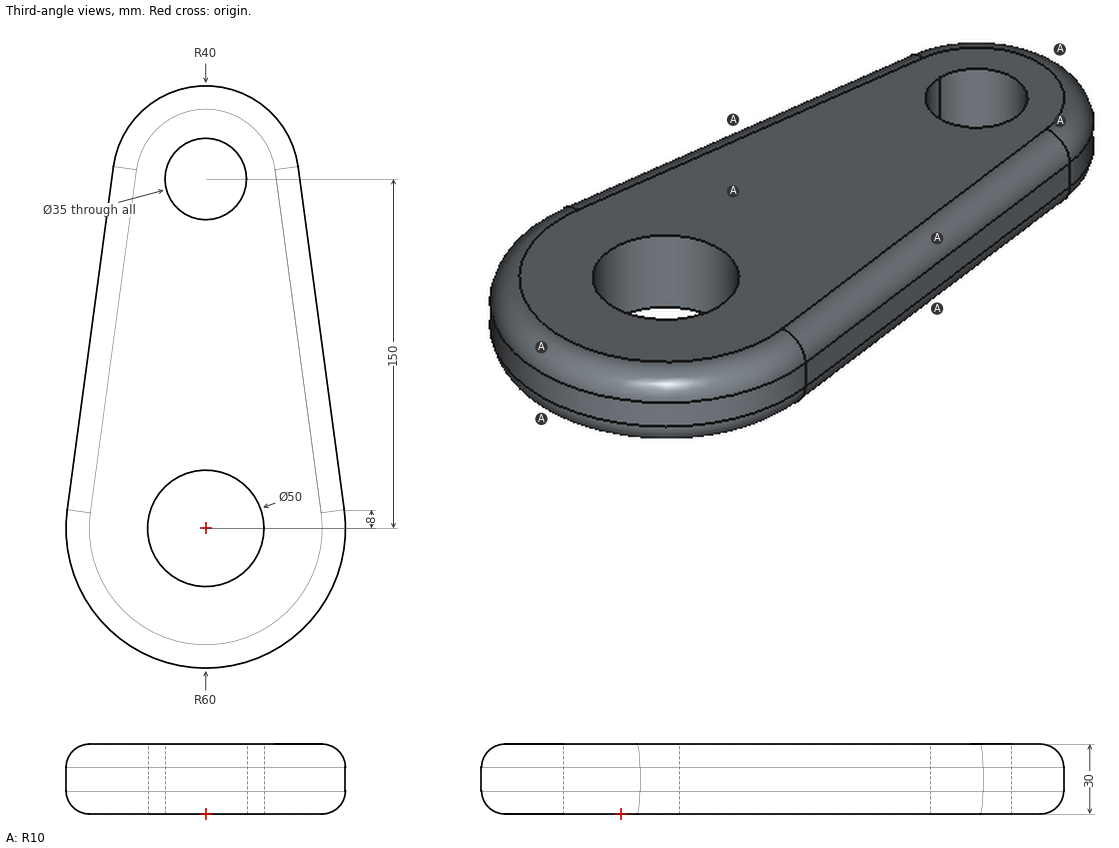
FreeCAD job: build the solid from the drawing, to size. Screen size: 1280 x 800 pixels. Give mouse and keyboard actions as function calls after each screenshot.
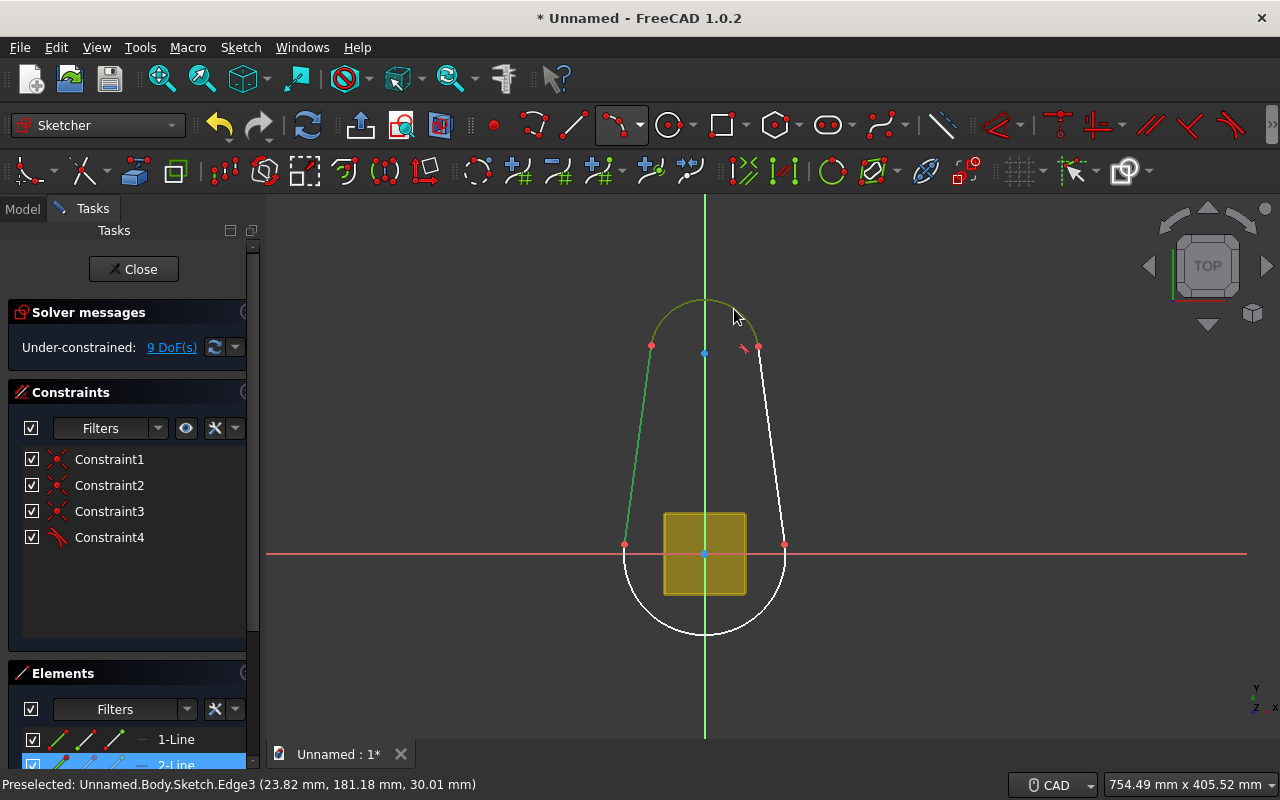
click(1232, 126)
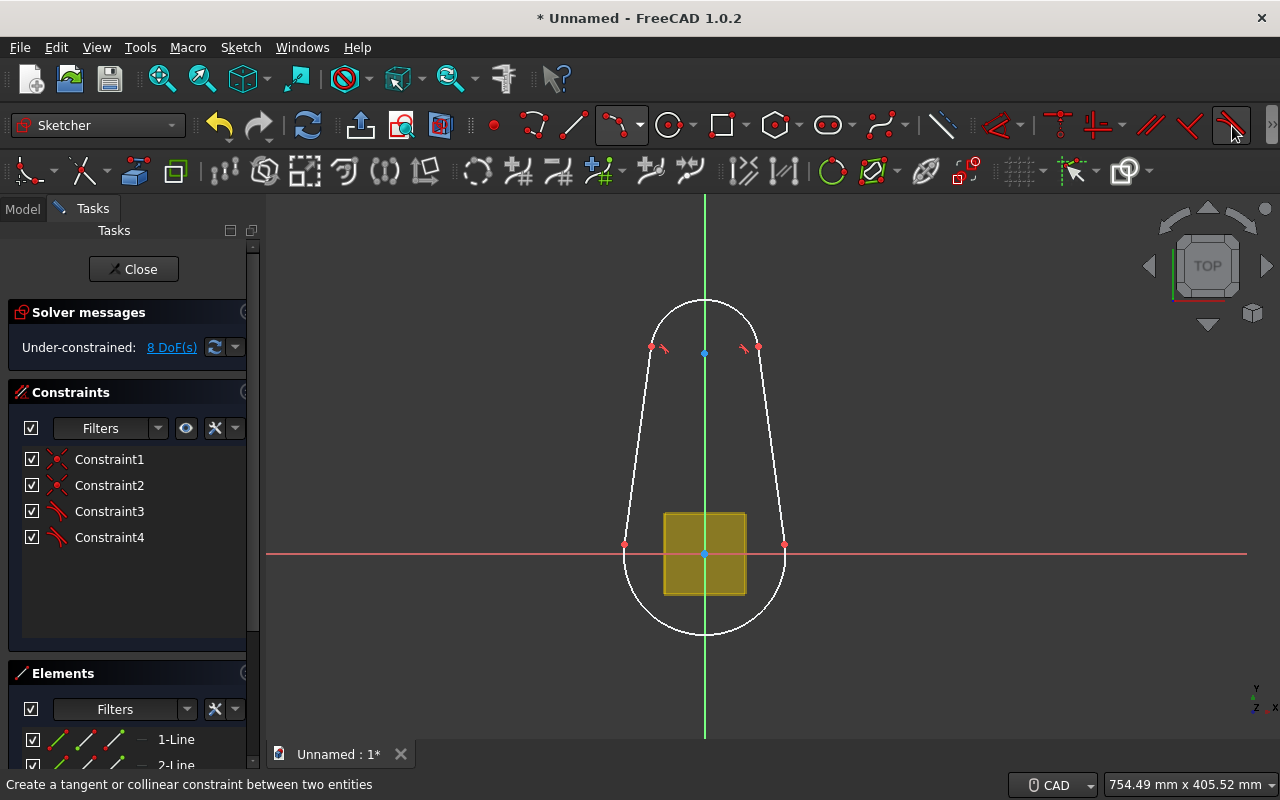
drag(695, 544, 715, 564)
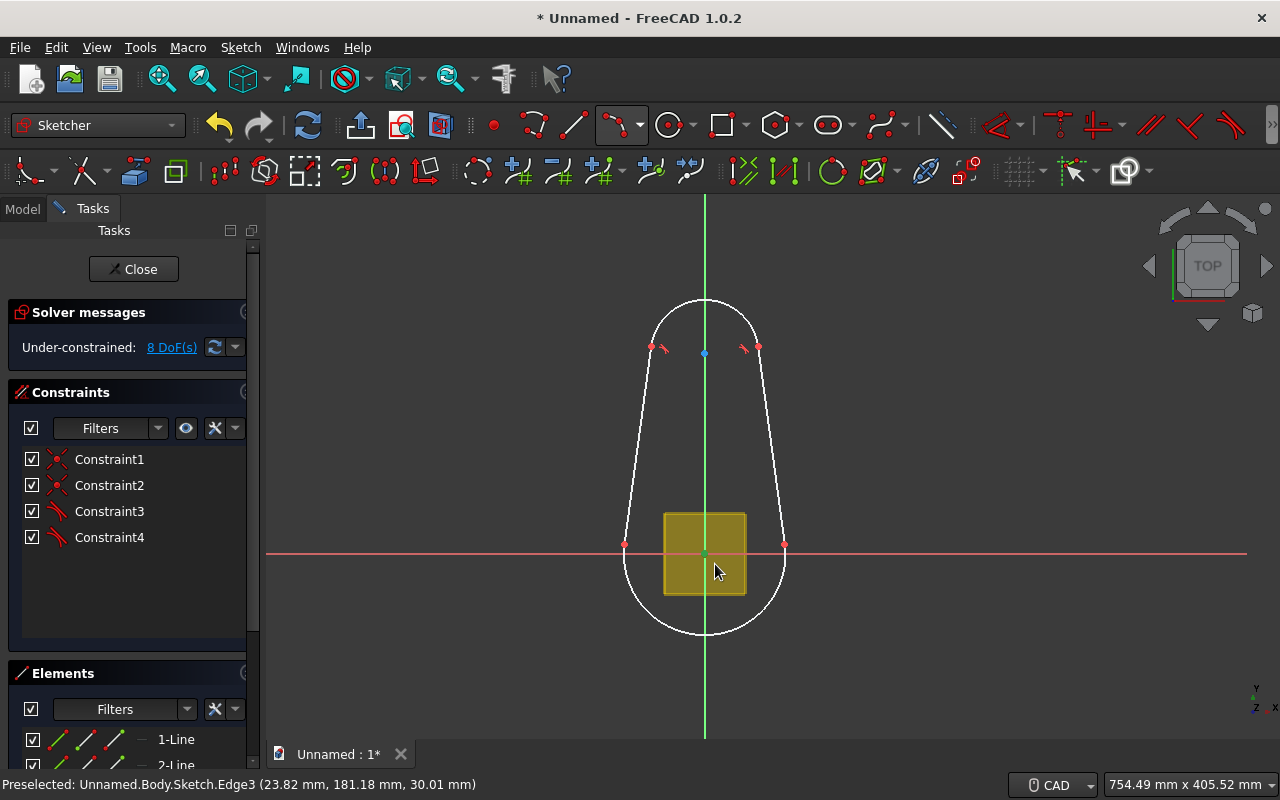
click(1058, 126)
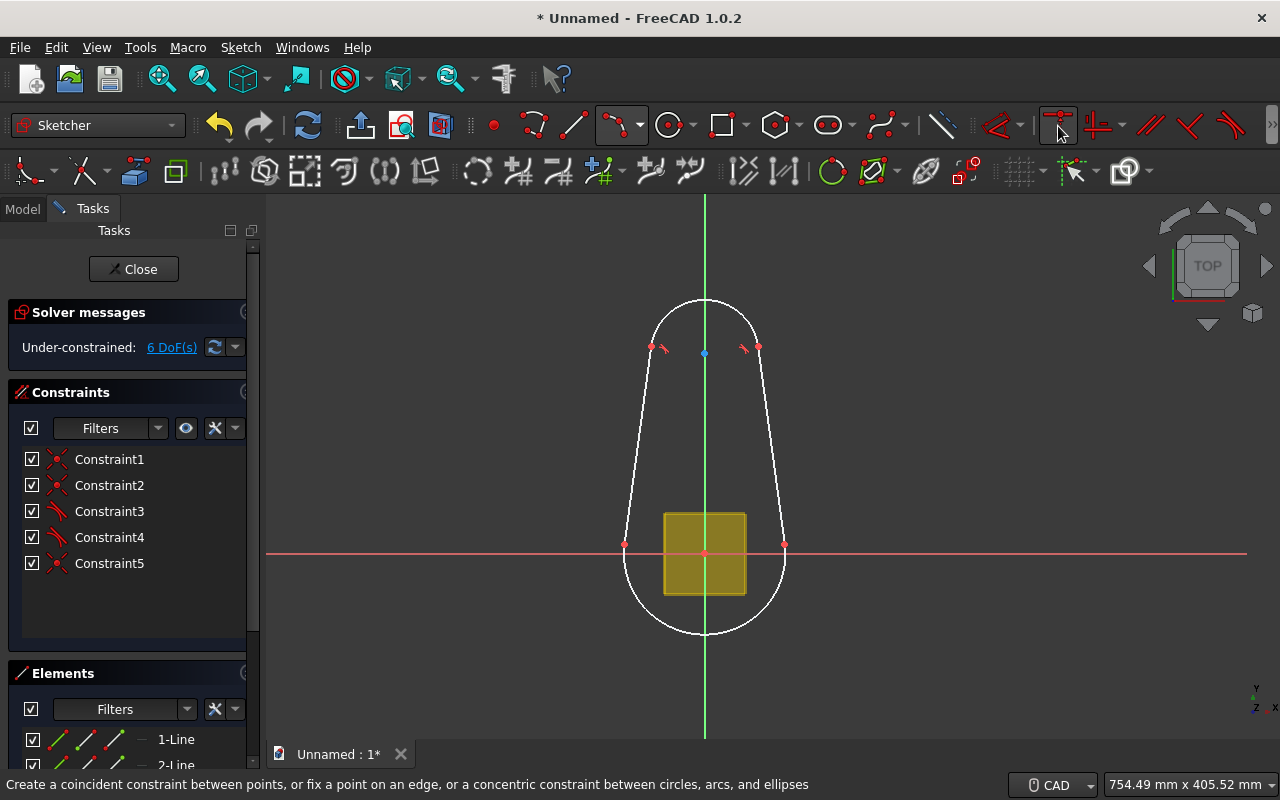
click(705, 354)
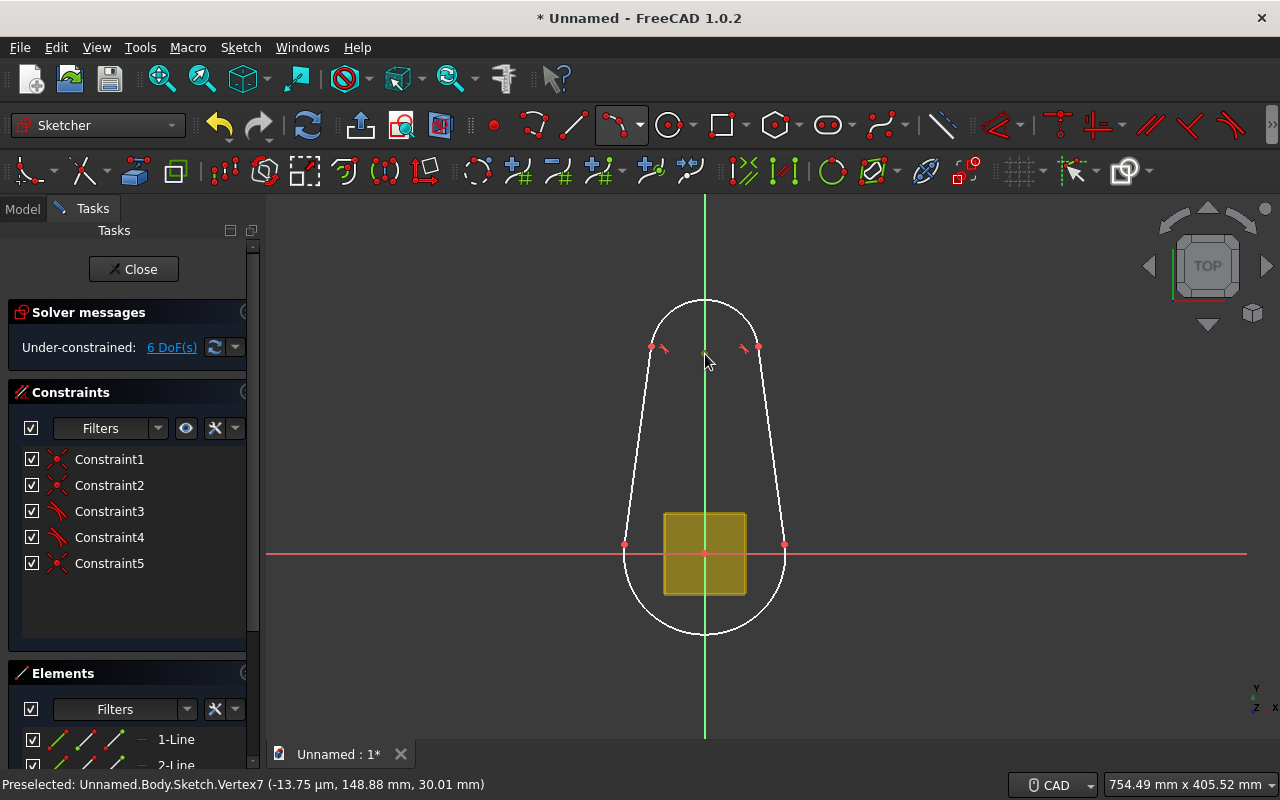
click(705, 676)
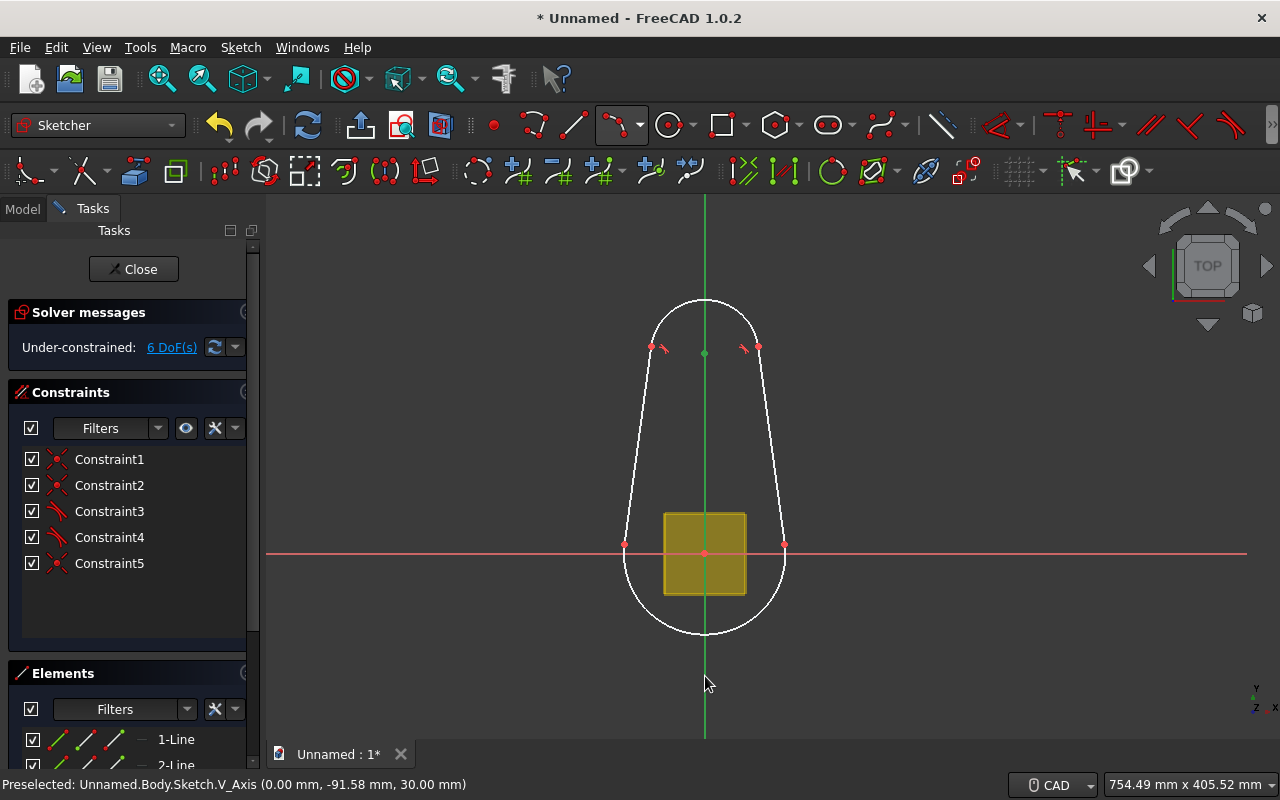
click(1058, 126)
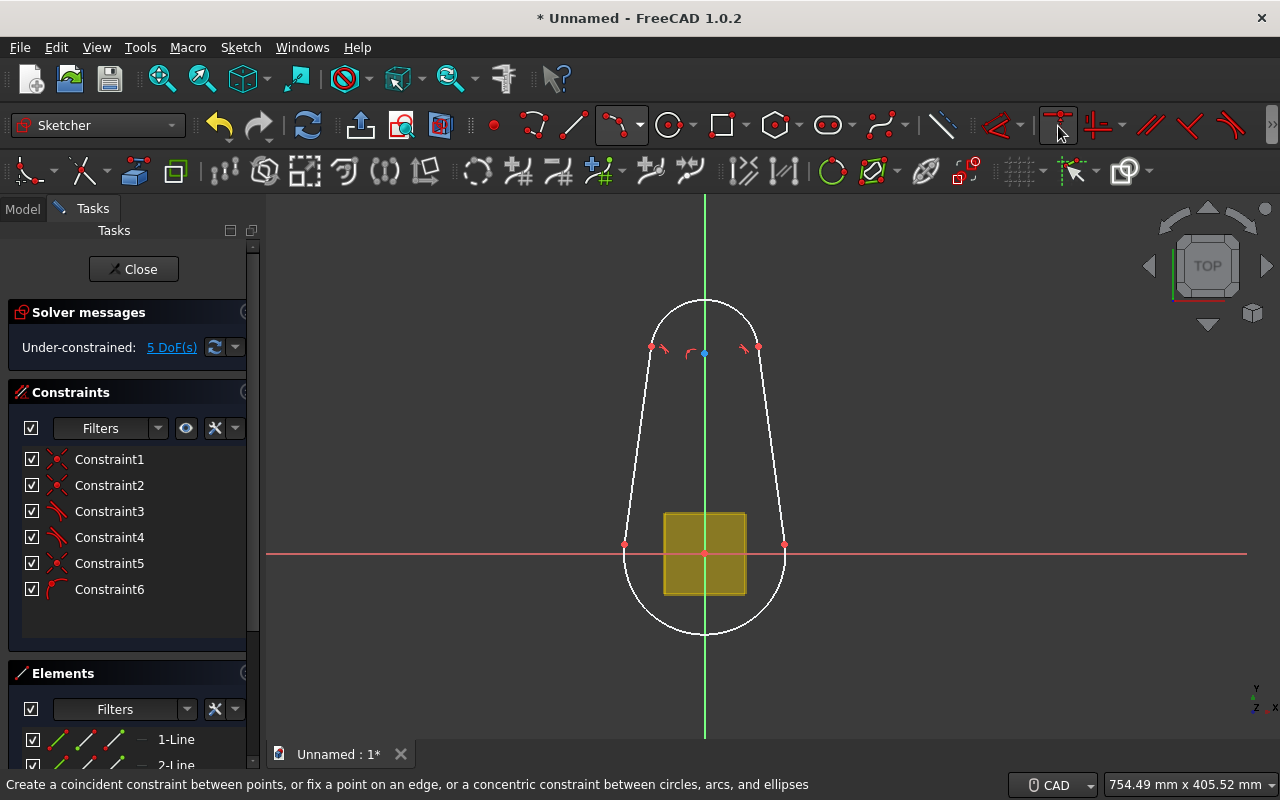
click(734, 309)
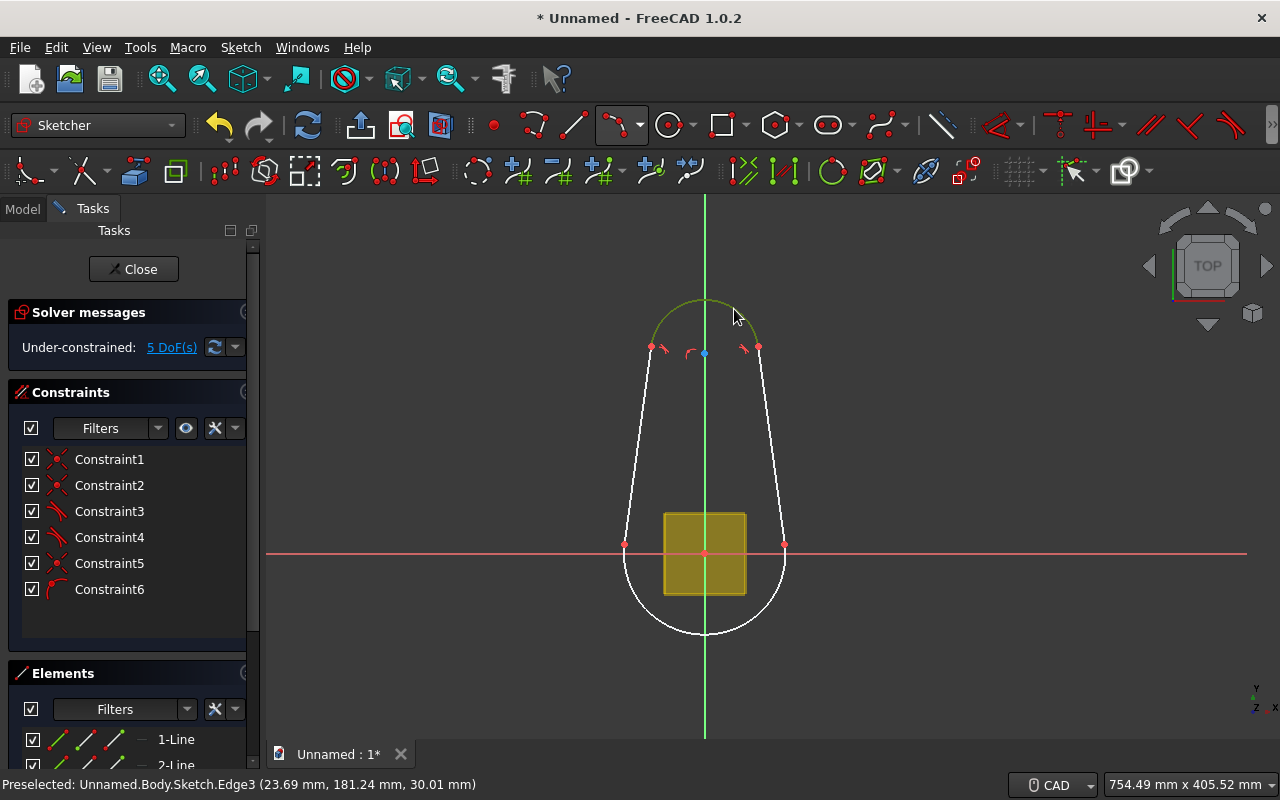
click(1022, 126)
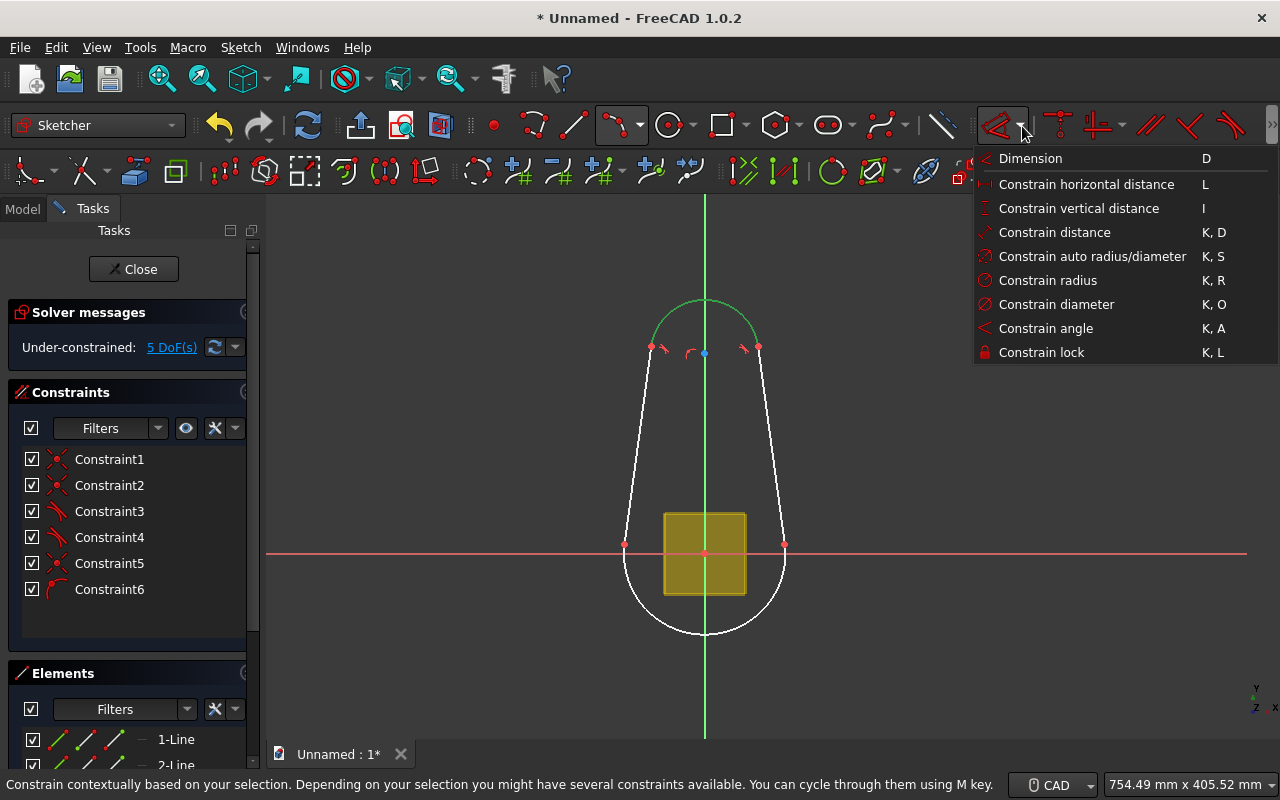
click(1126, 280)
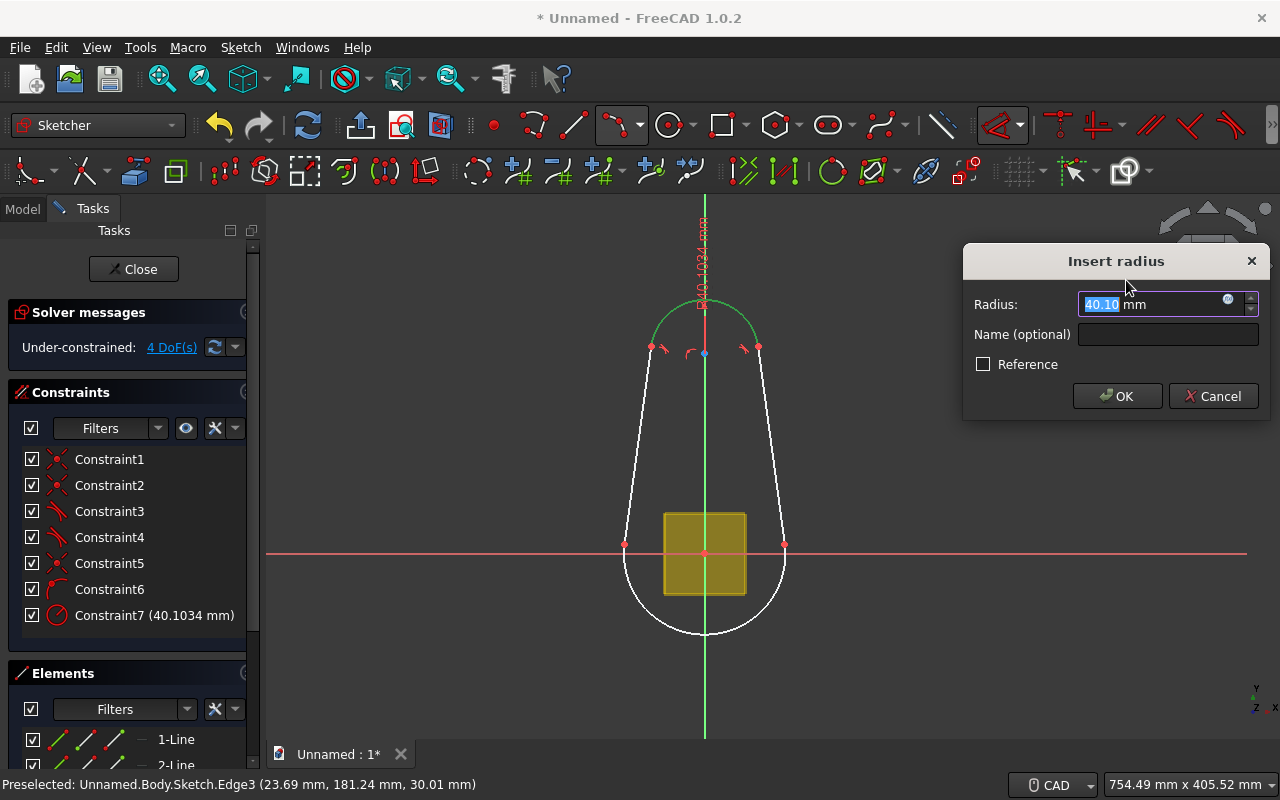
text(40)
key(Return)